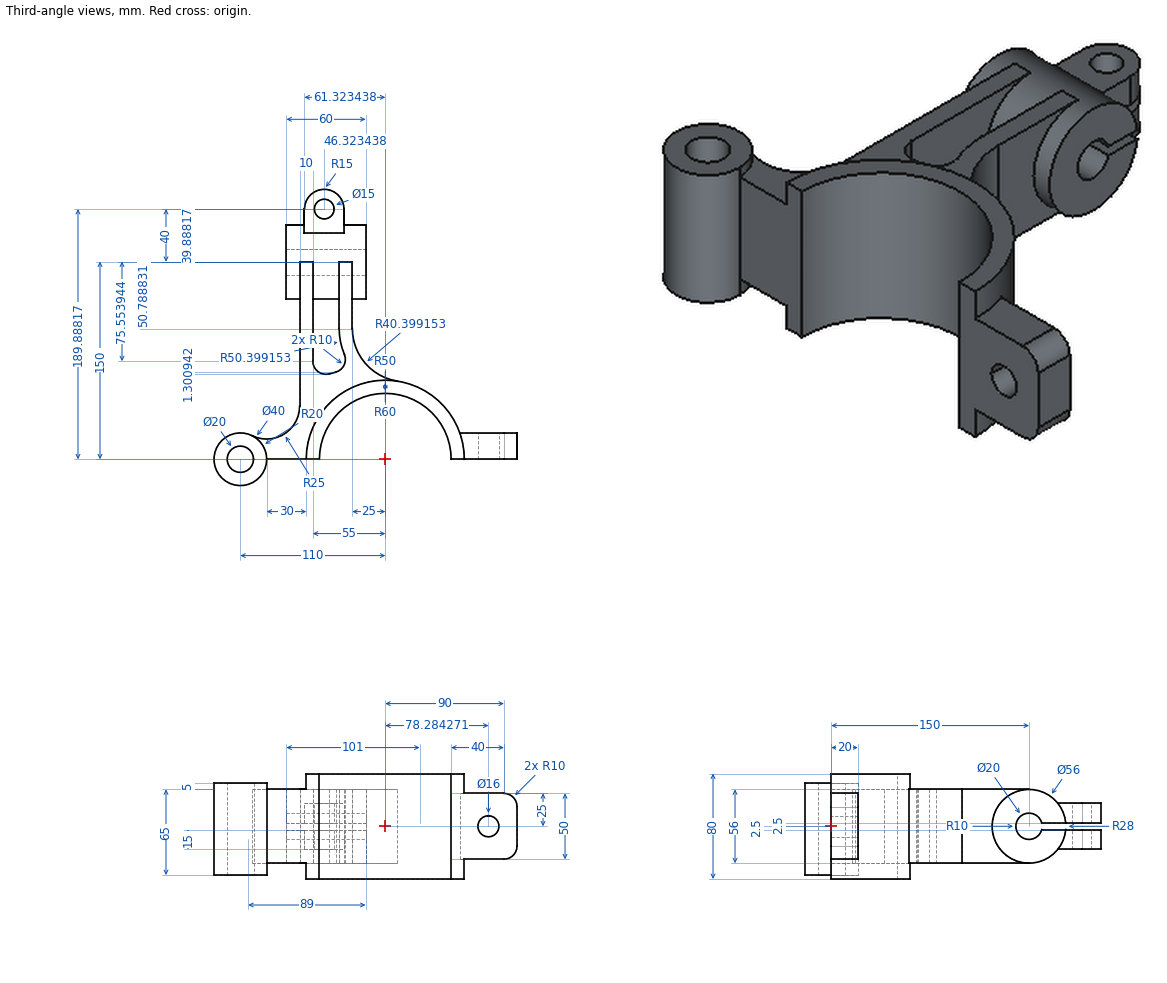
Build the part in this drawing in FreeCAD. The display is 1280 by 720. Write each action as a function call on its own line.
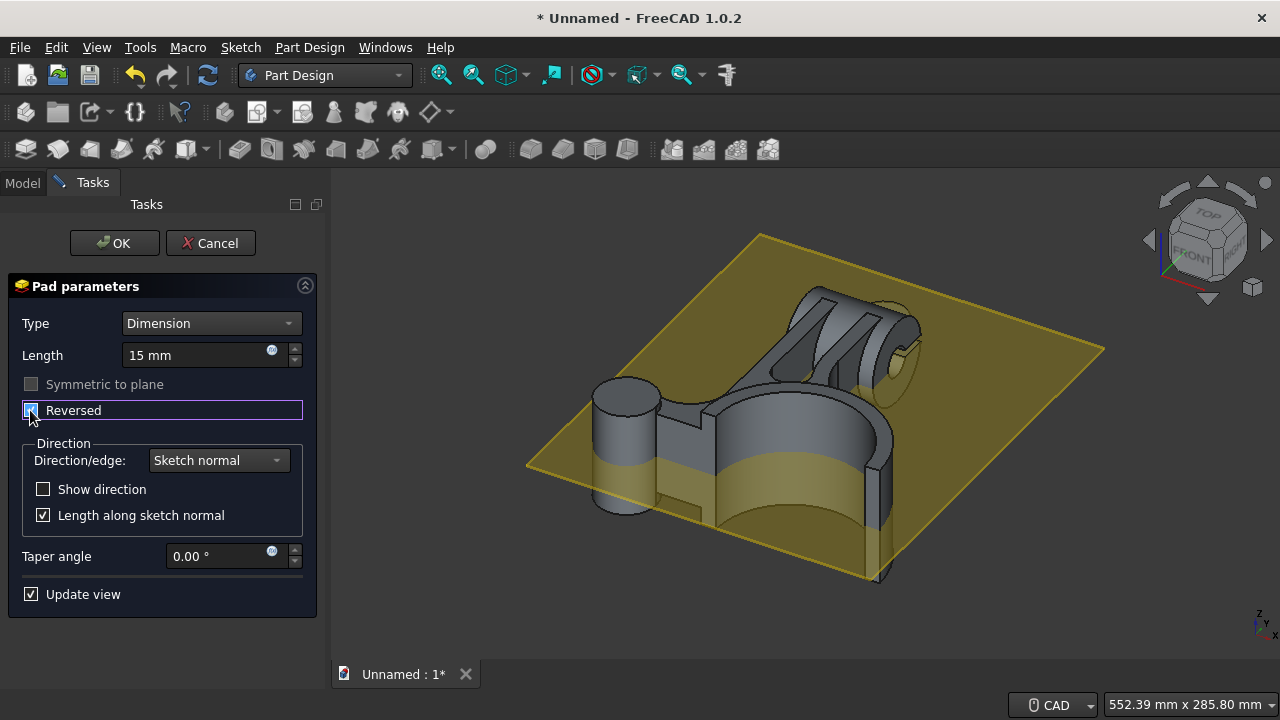
click(115, 243)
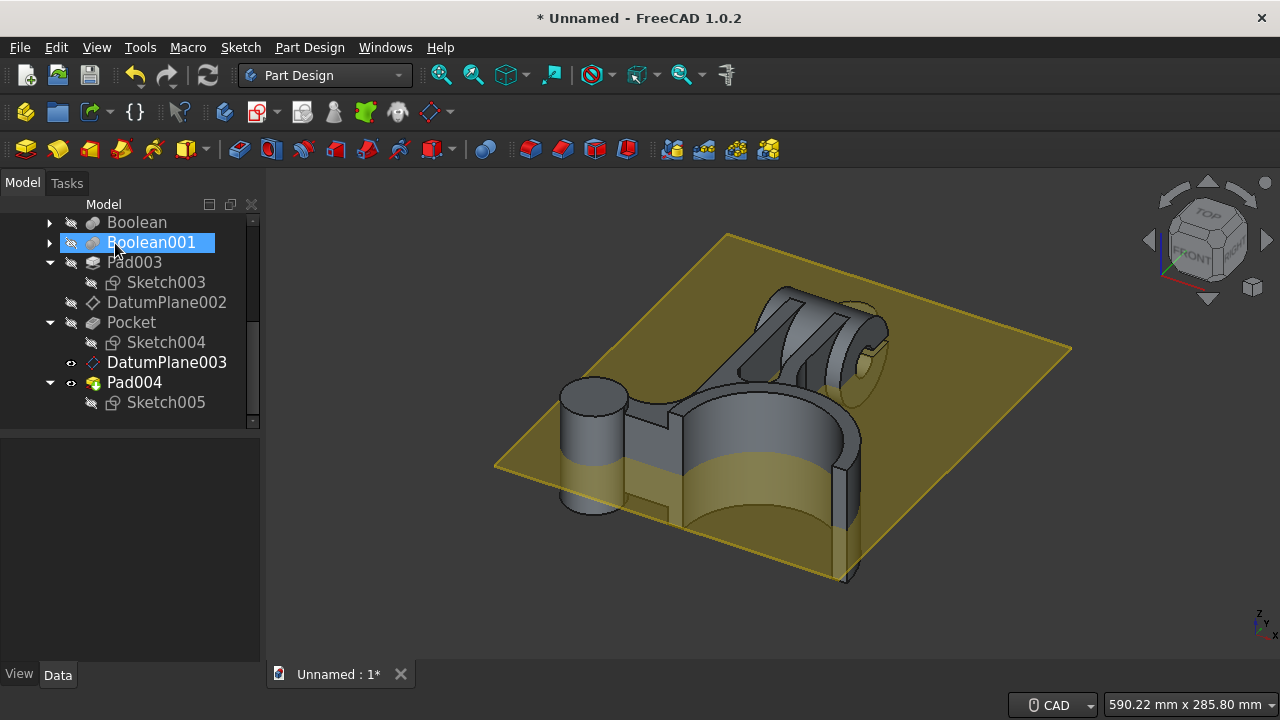
click(116, 363)
key(space)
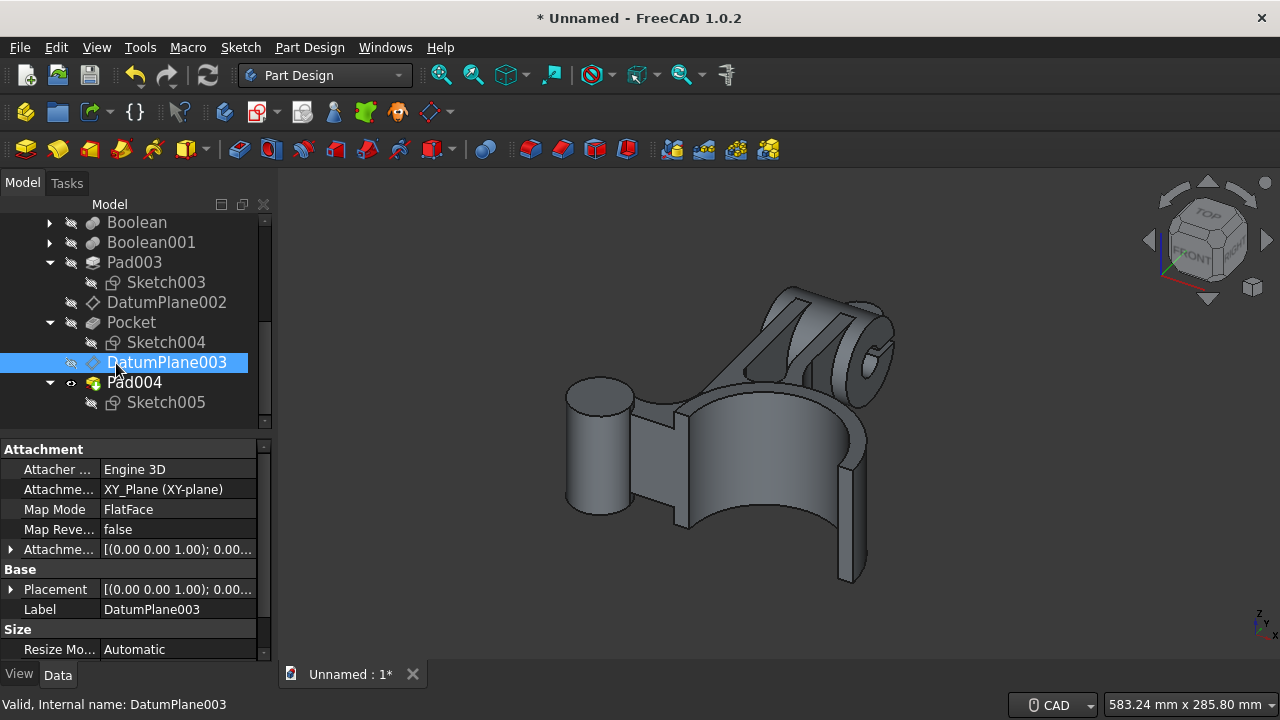
click(116, 383)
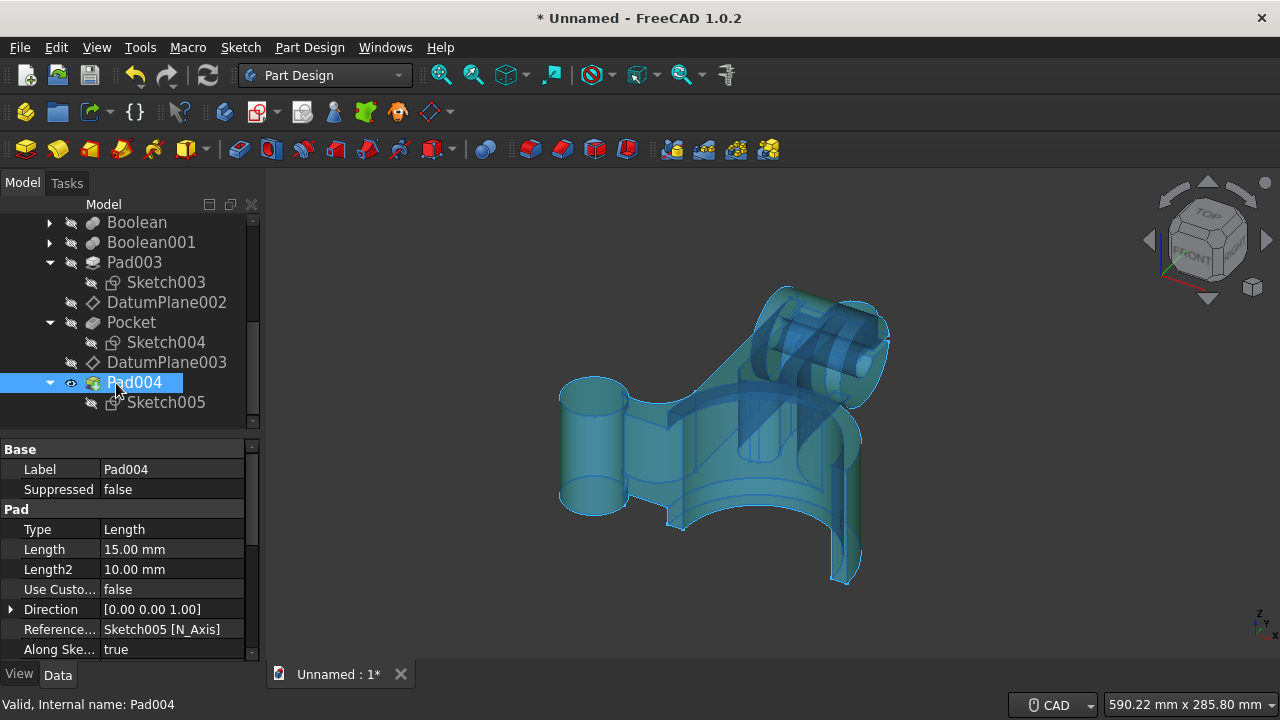
click(672, 150)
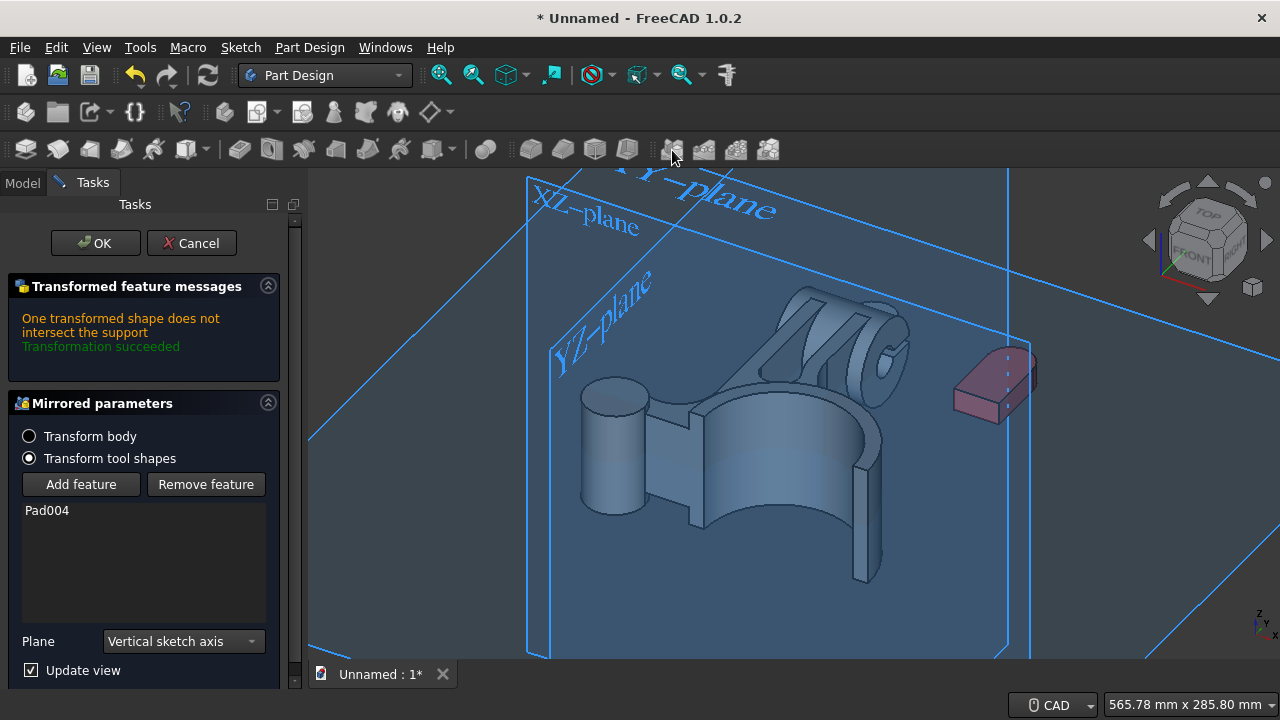
click(184, 642)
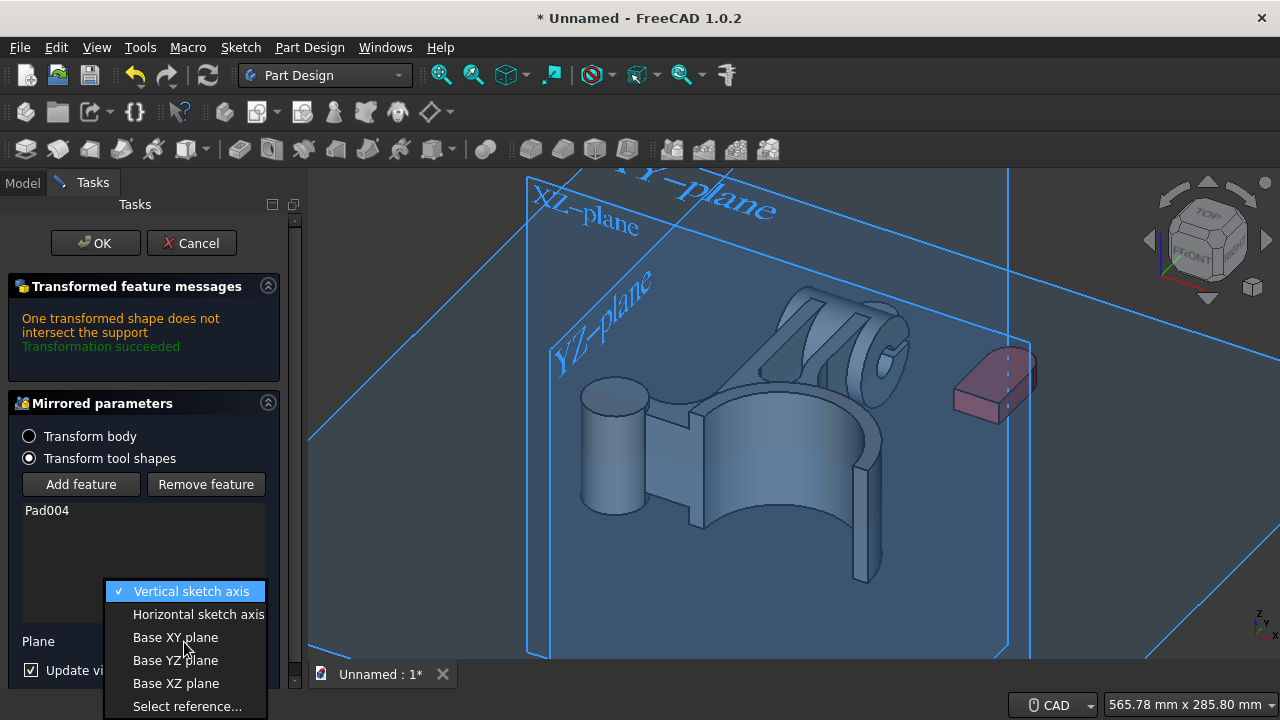
click(184, 638)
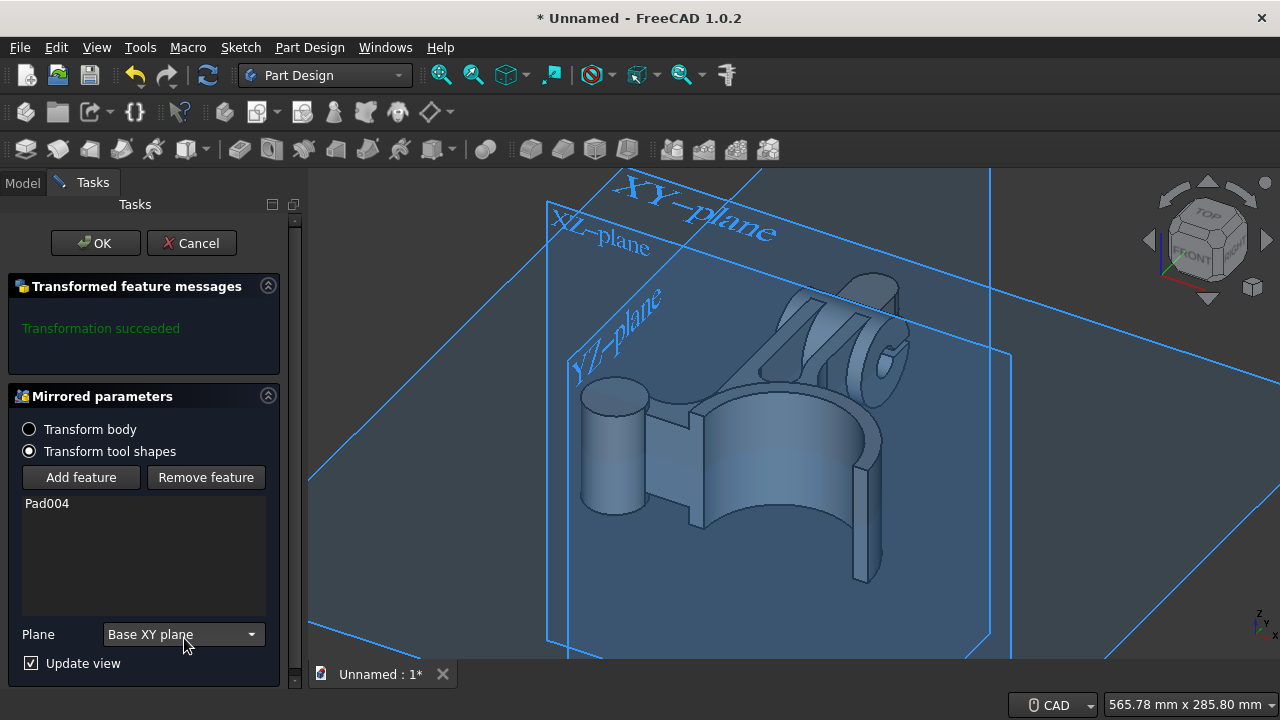
click(96, 243)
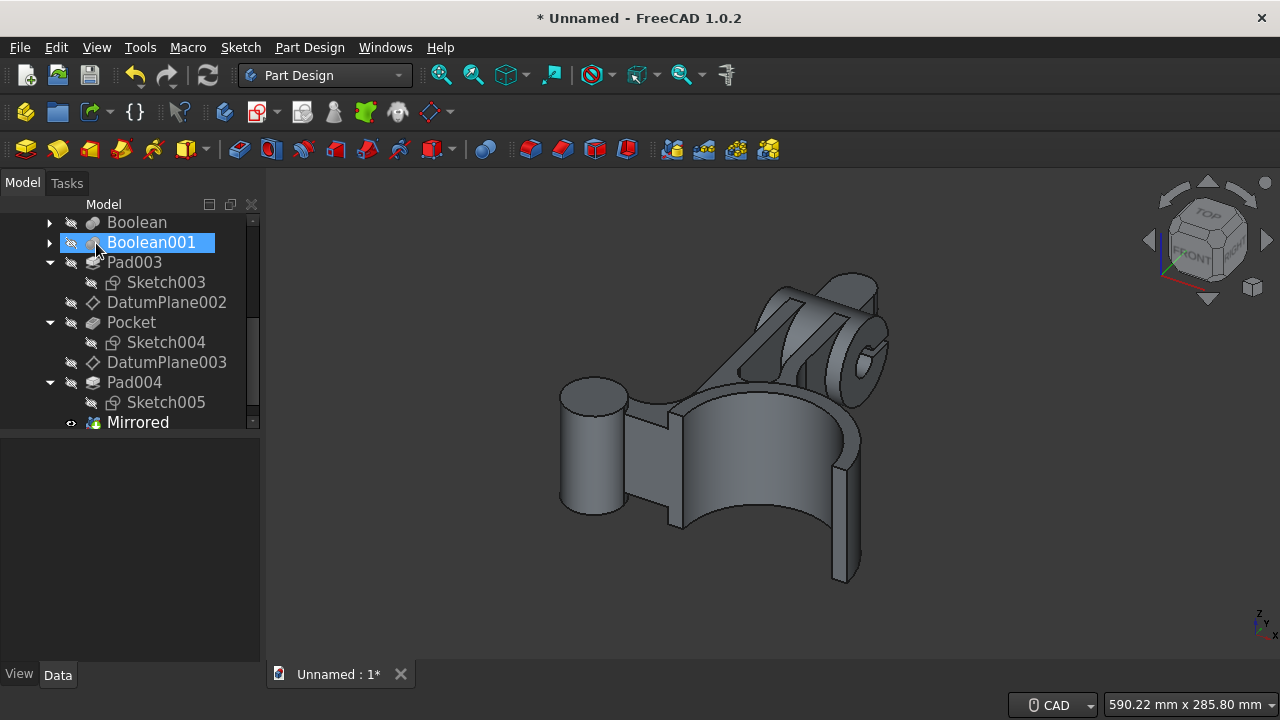
click(851, 386)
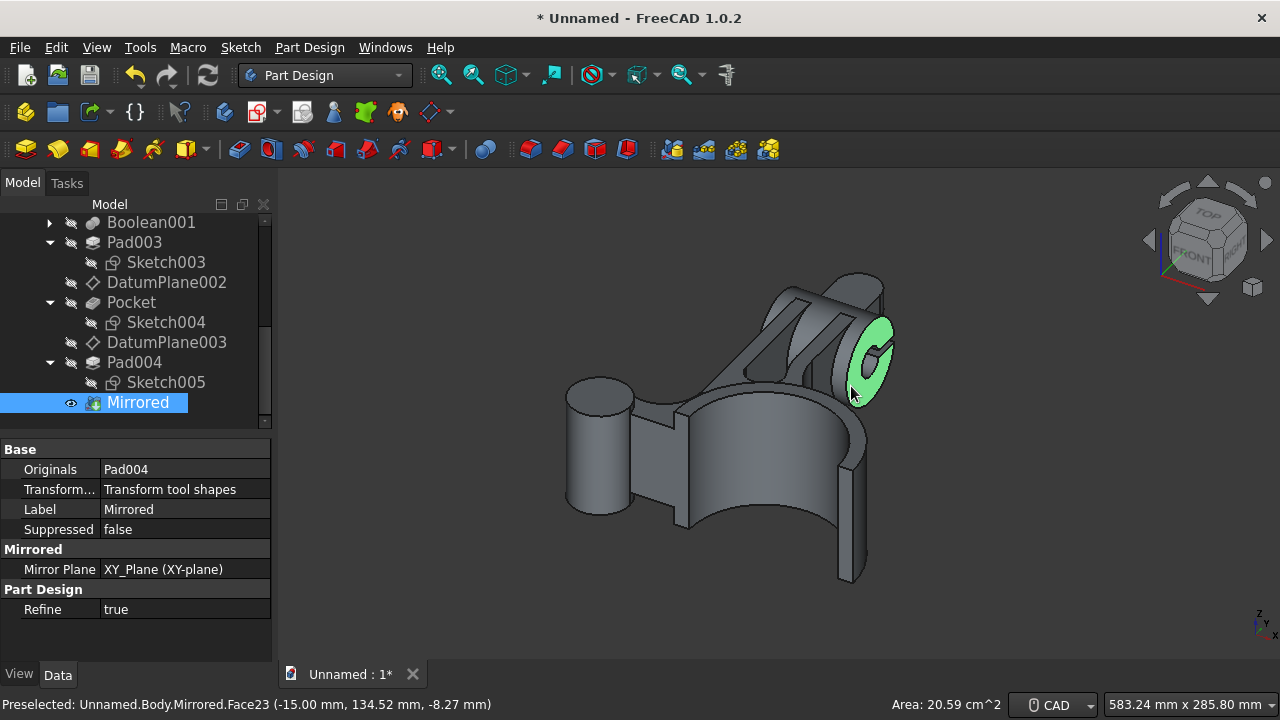
click(258, 112)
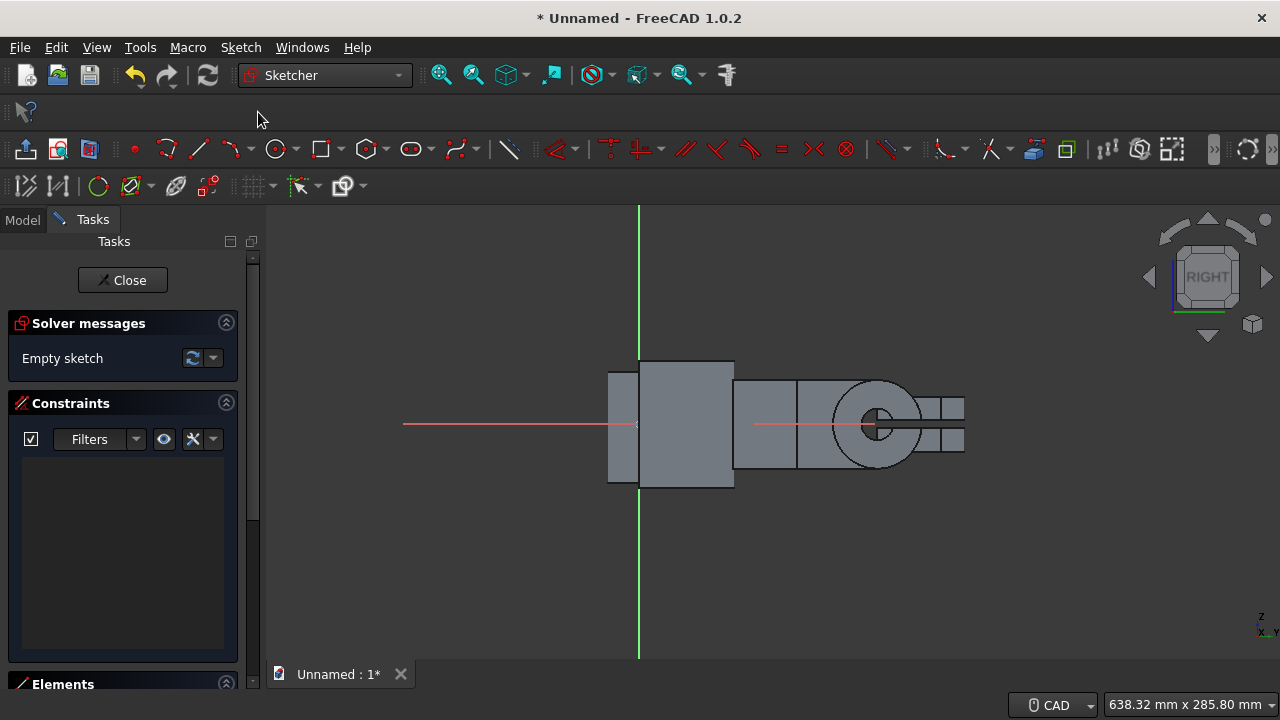
key(q)
key(s)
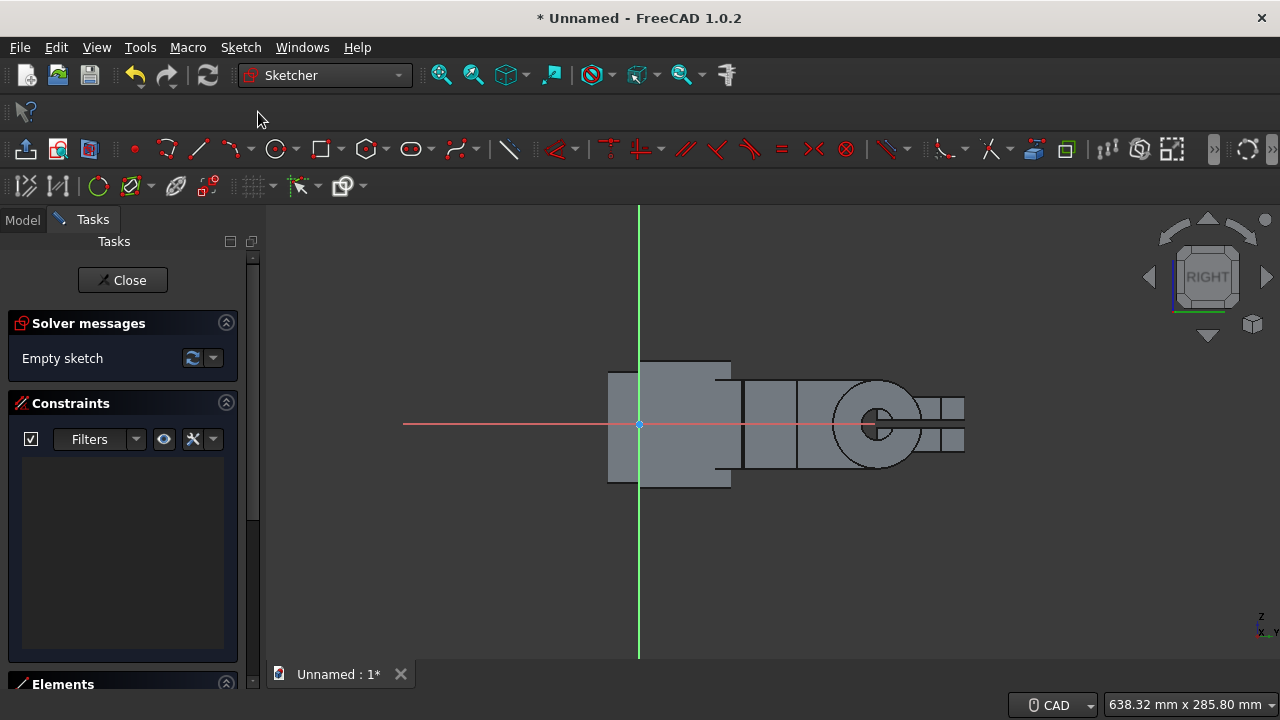
scroll(899, 423, up, 11)